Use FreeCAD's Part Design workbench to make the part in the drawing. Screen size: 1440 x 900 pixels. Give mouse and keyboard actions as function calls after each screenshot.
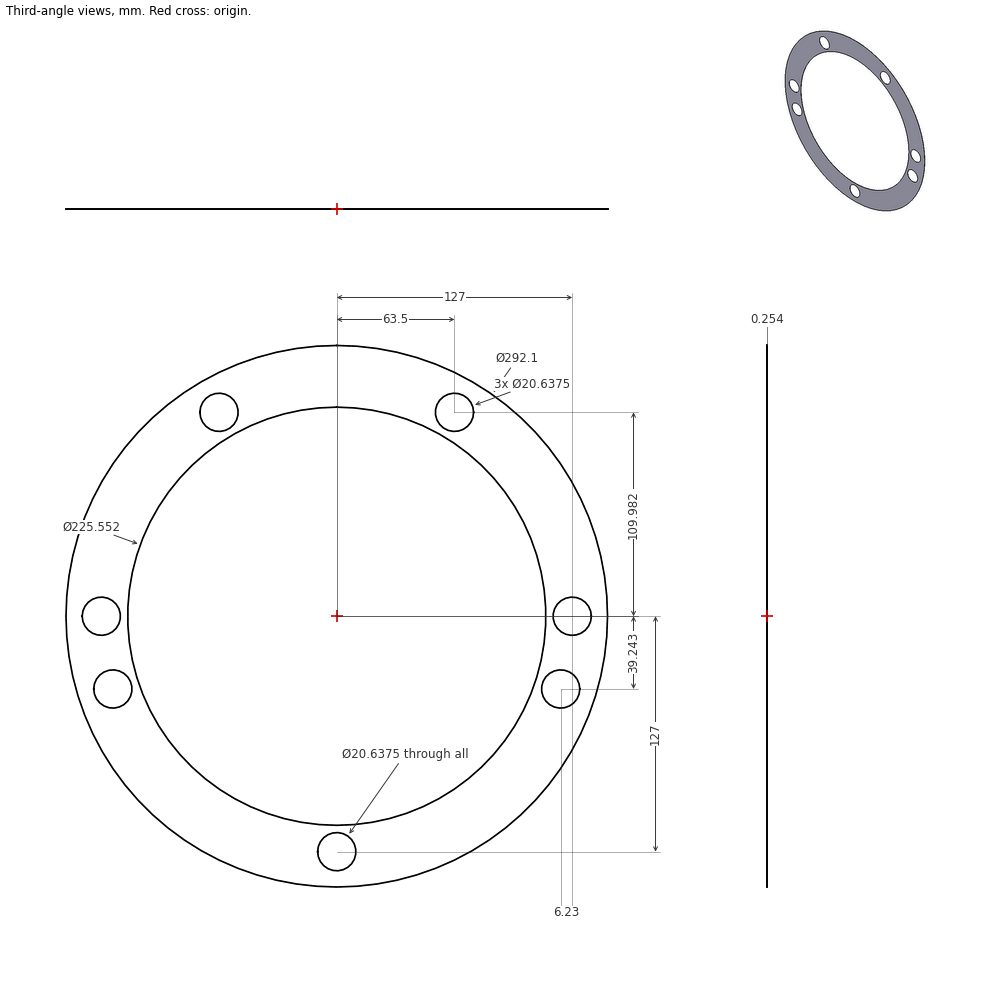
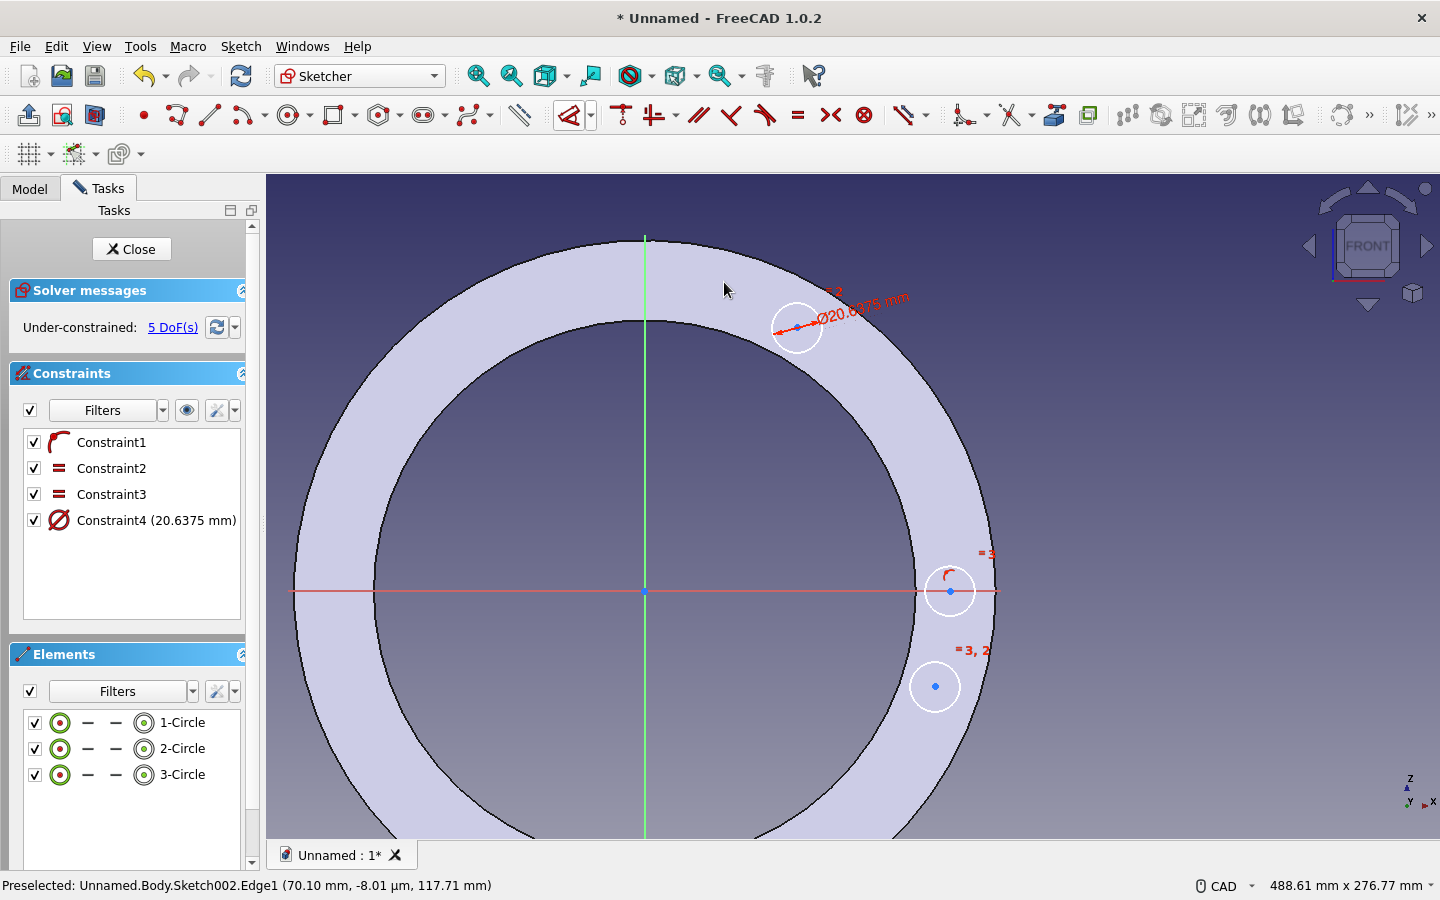
click(950, 591)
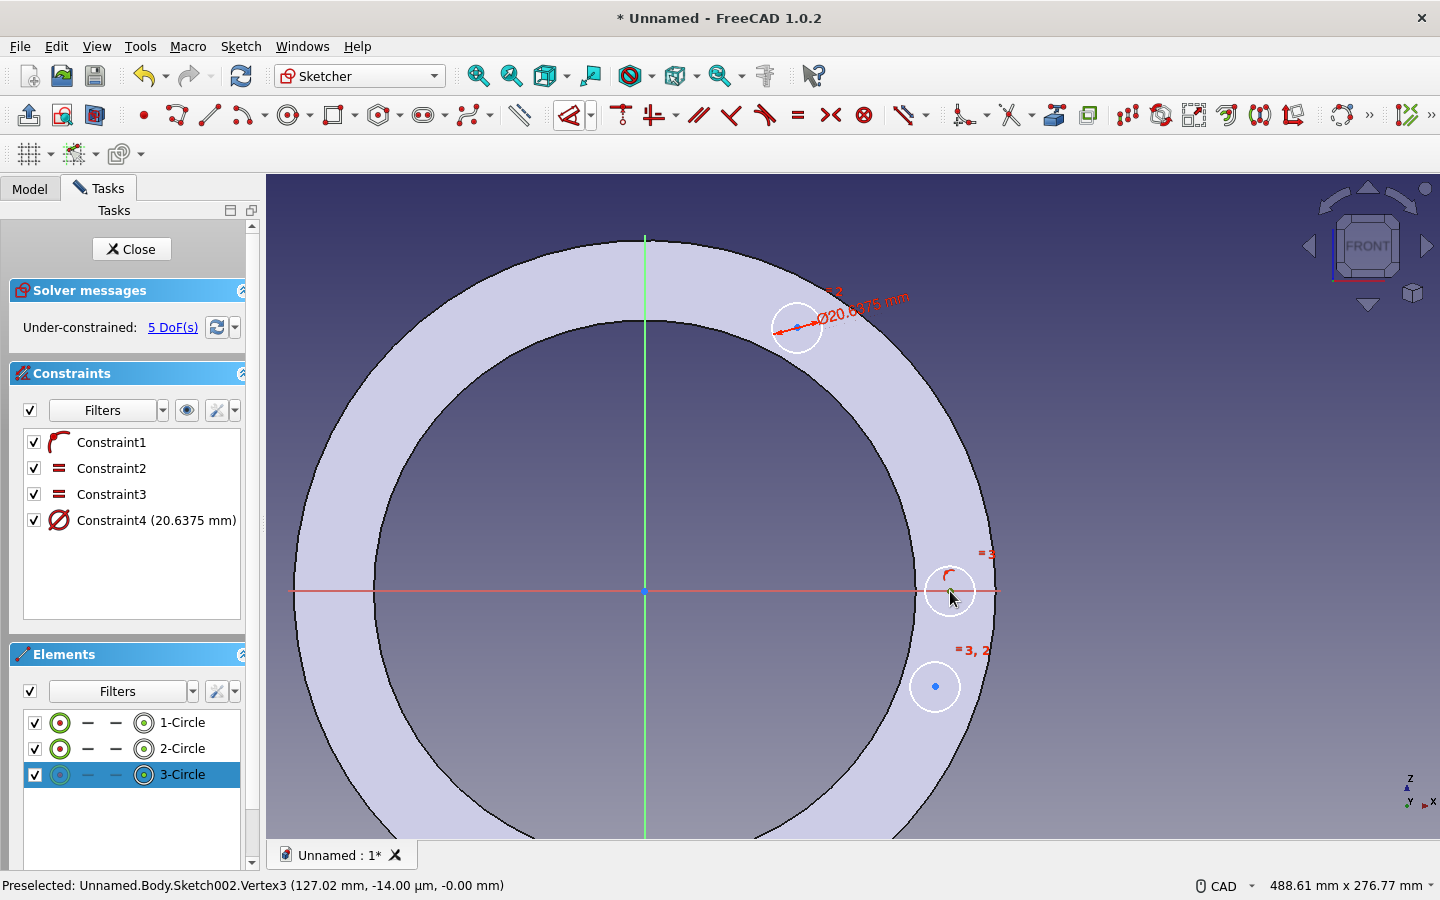
key(l)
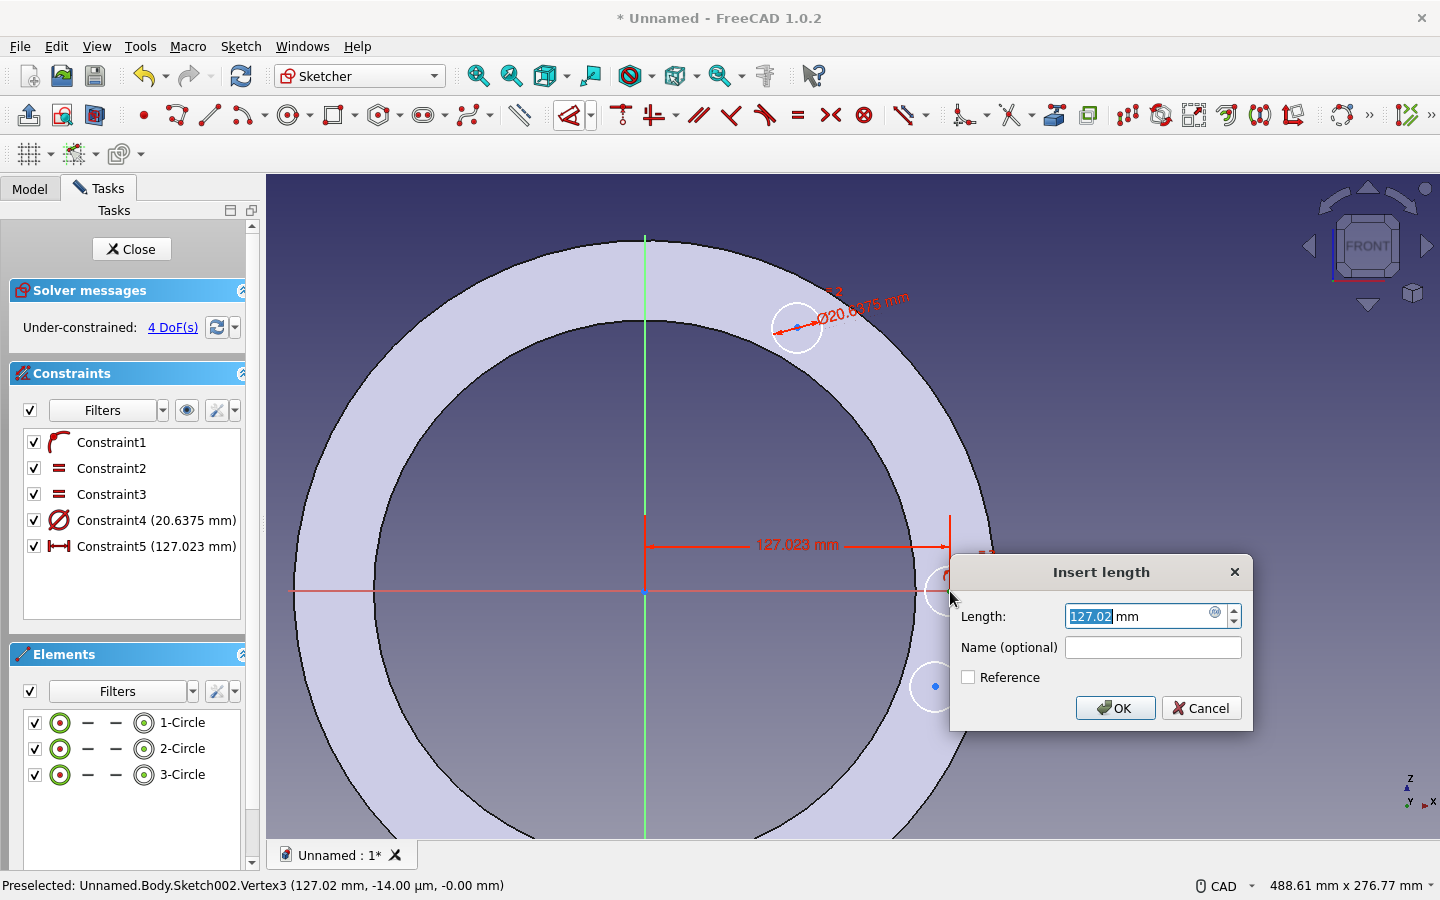
text(127)
key(Return)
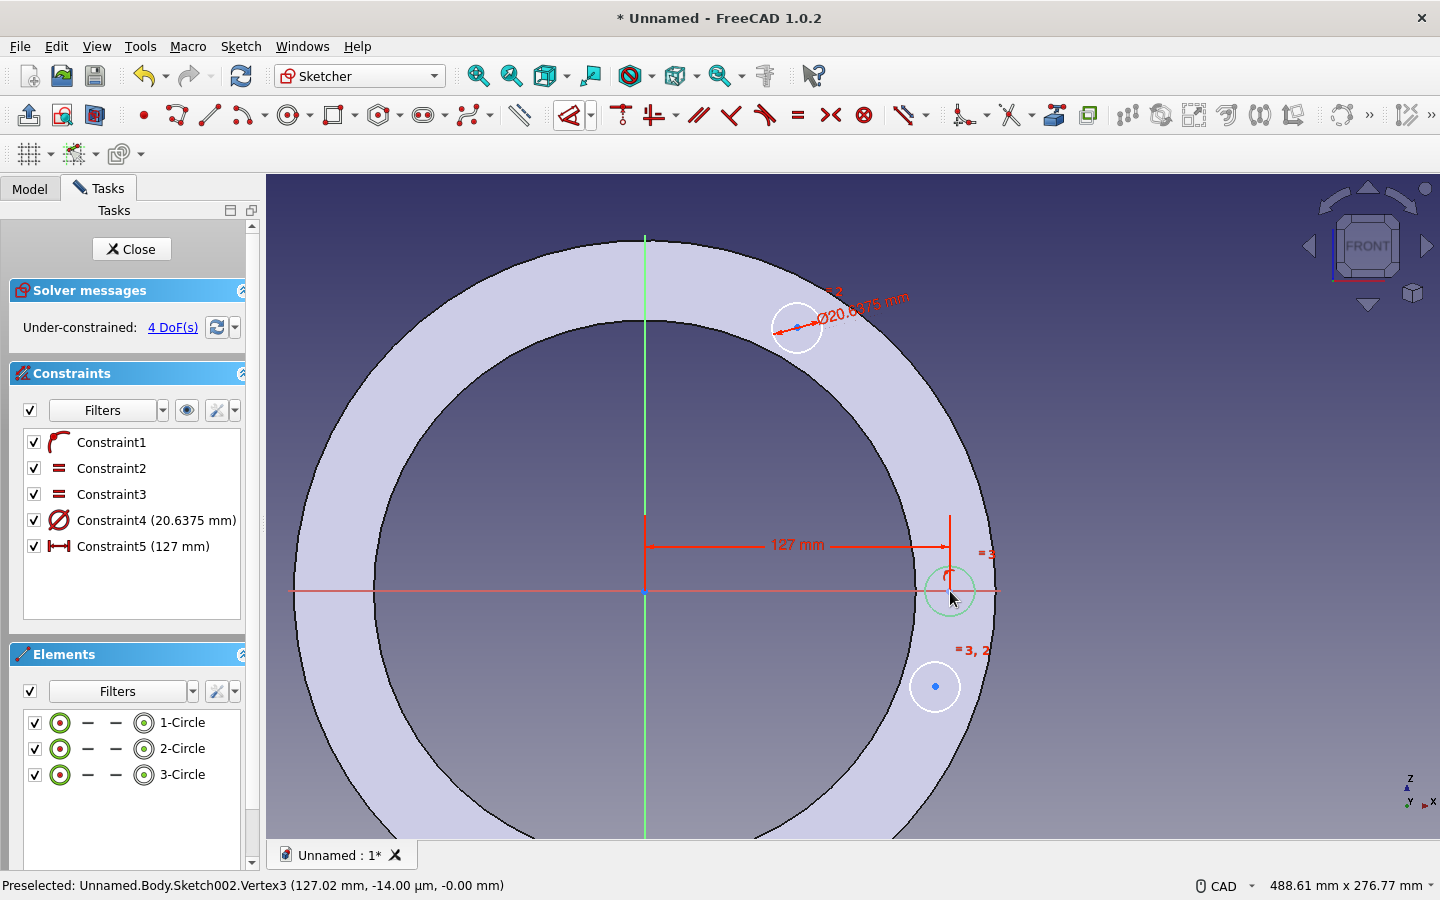
click(797, 328)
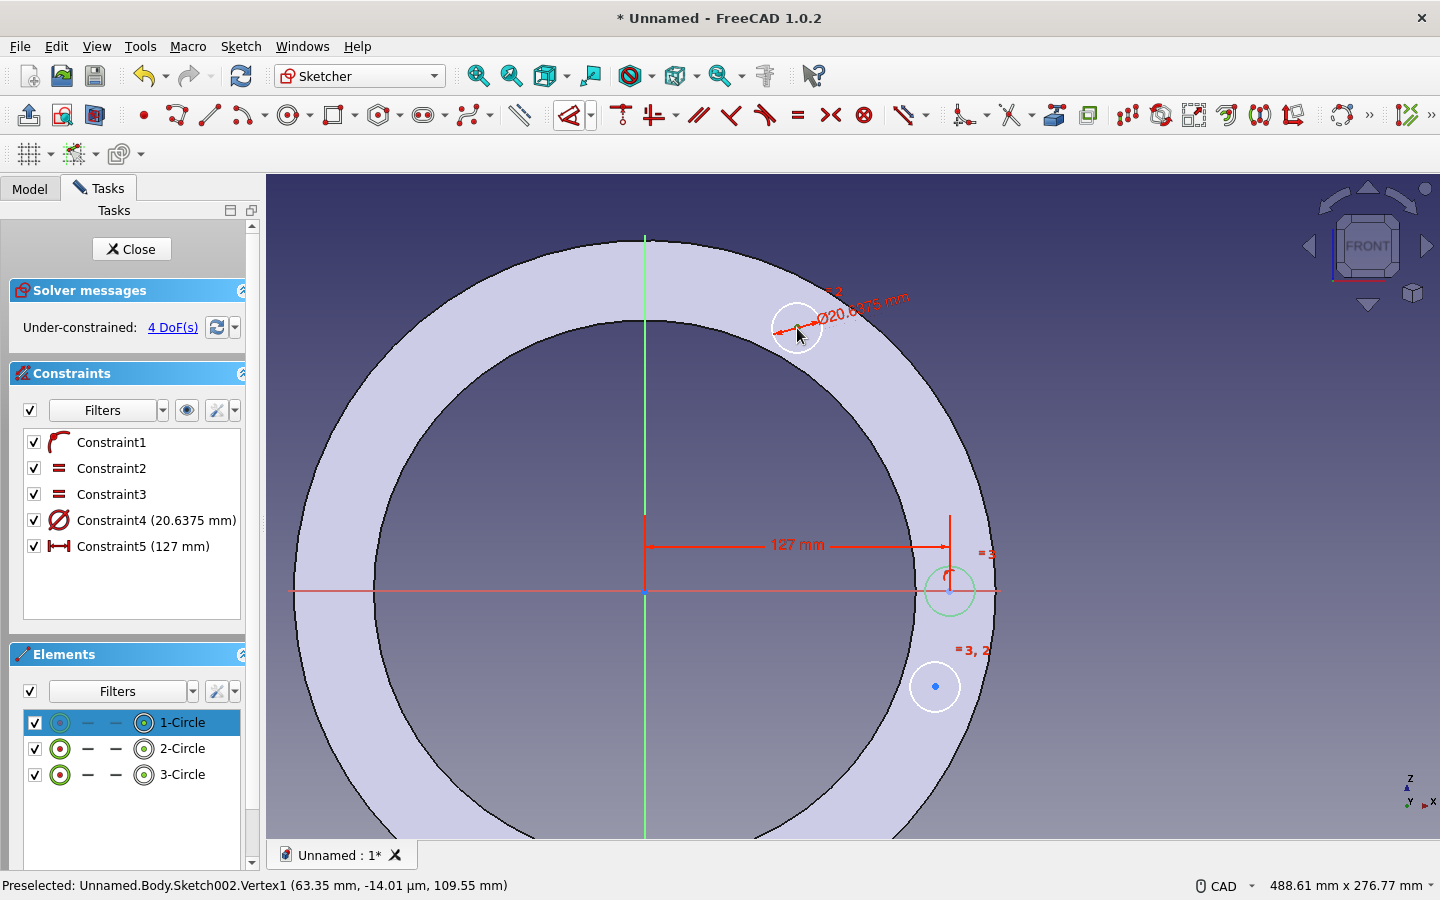
click(590, 116)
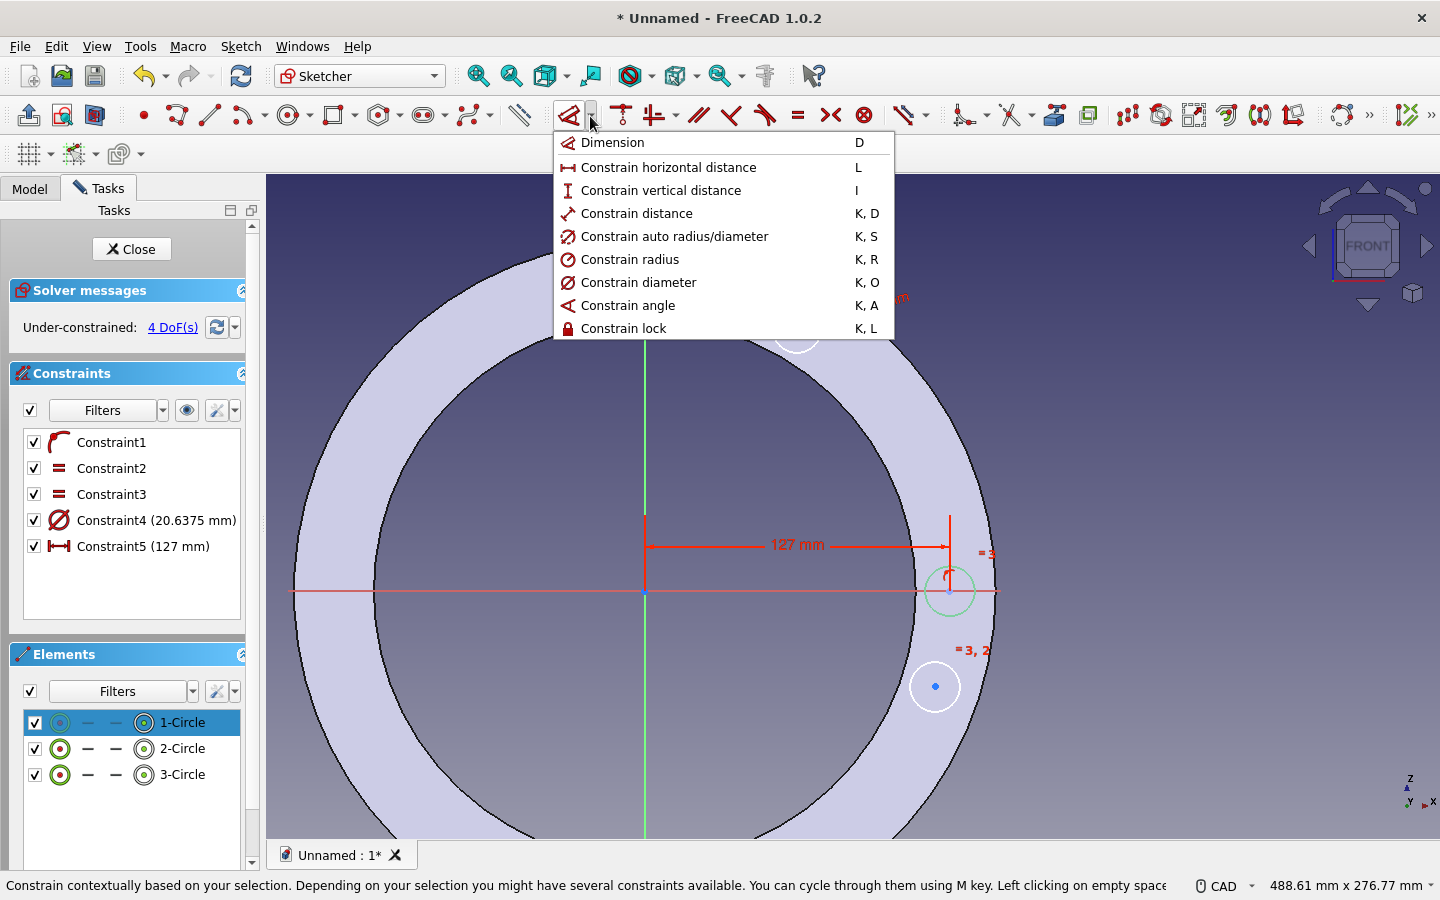
click(724, 168)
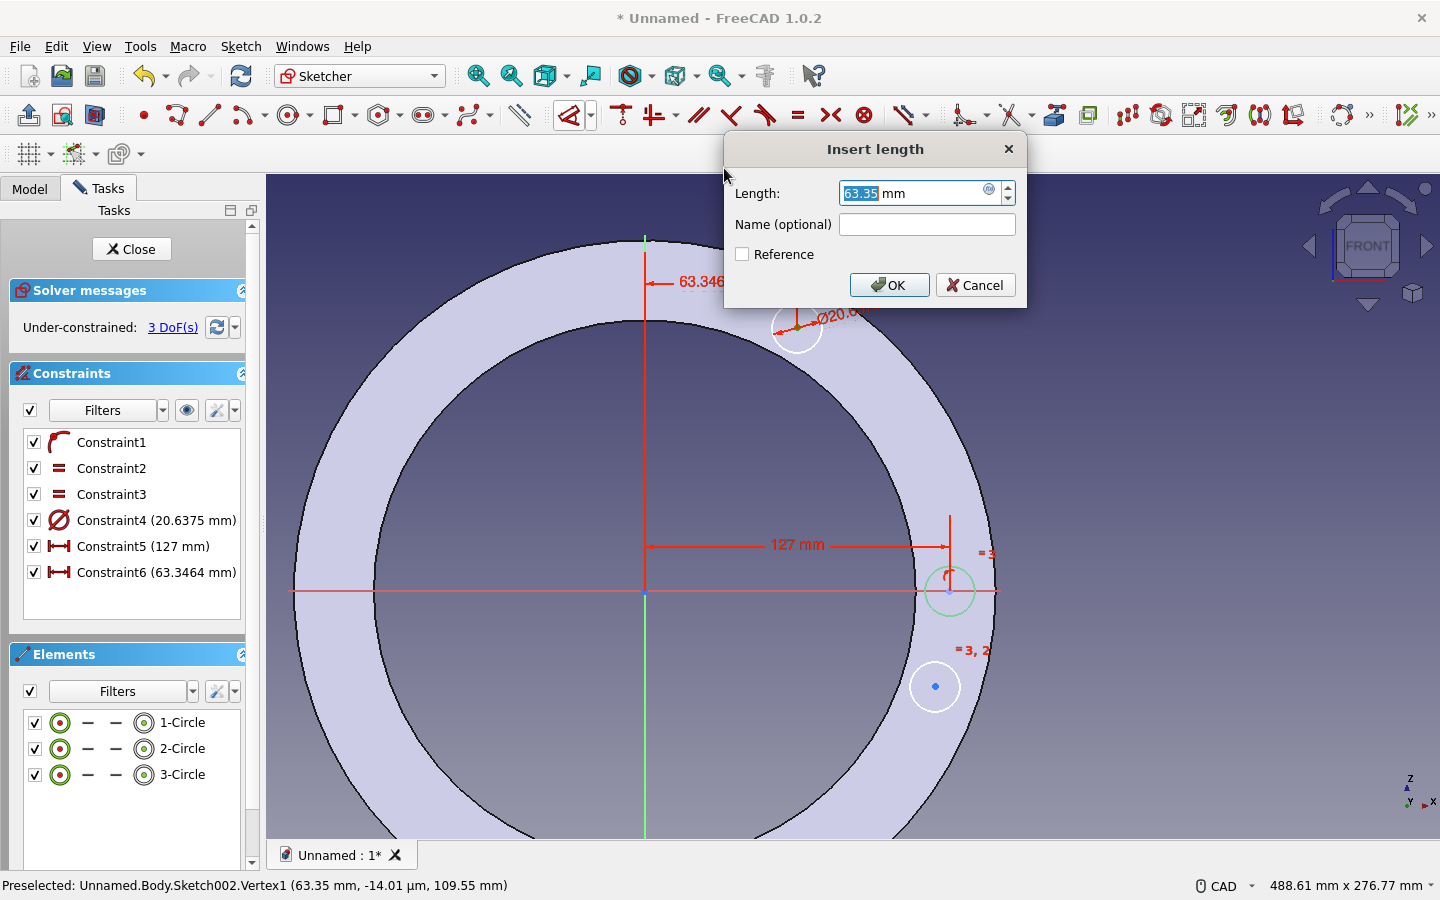
text(63.5)
key(Return)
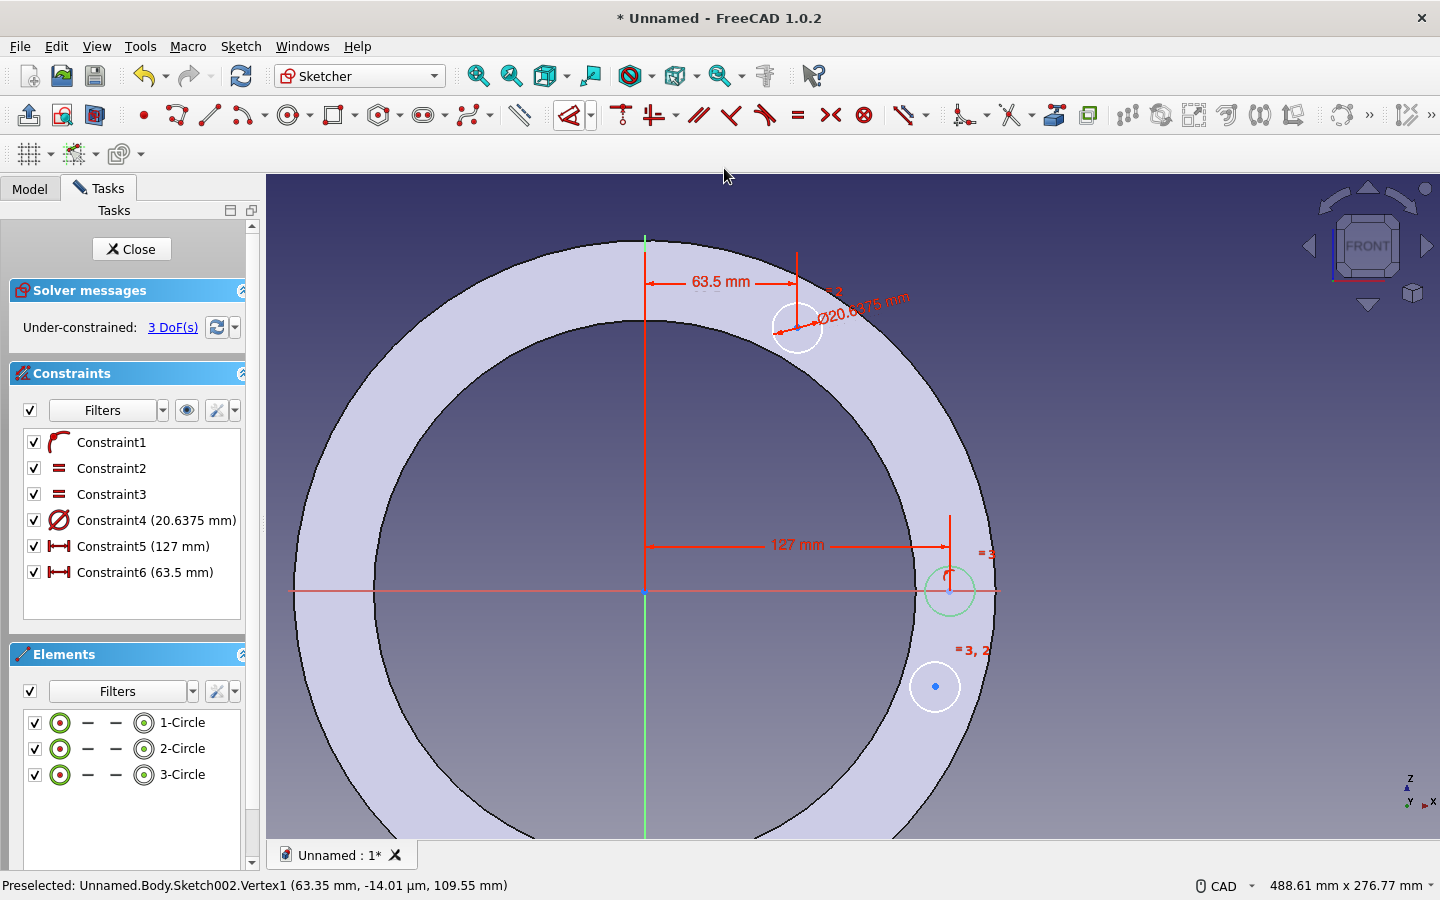
scroll(935, 687, up, 5)